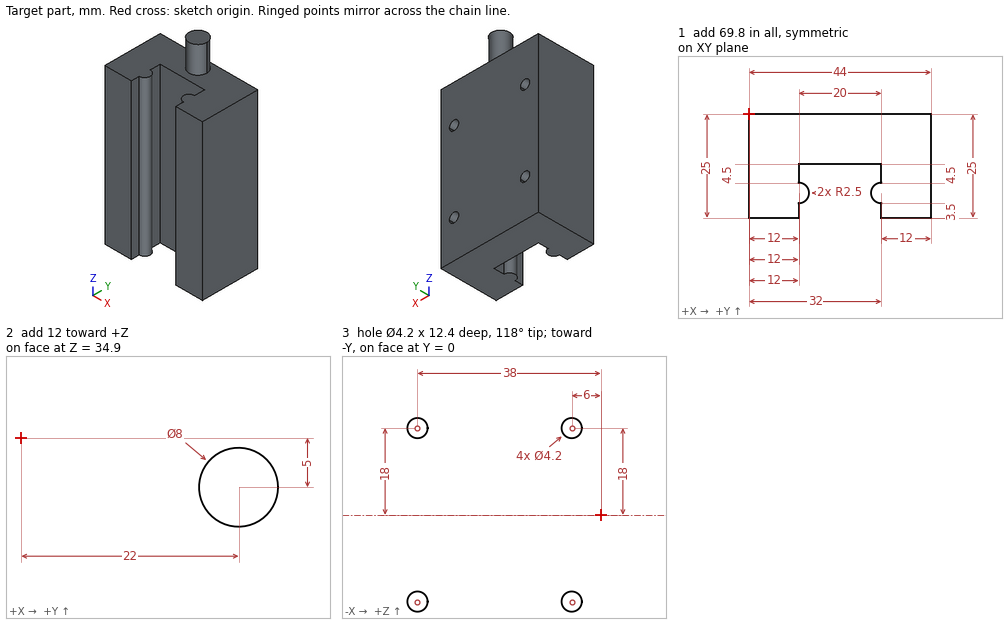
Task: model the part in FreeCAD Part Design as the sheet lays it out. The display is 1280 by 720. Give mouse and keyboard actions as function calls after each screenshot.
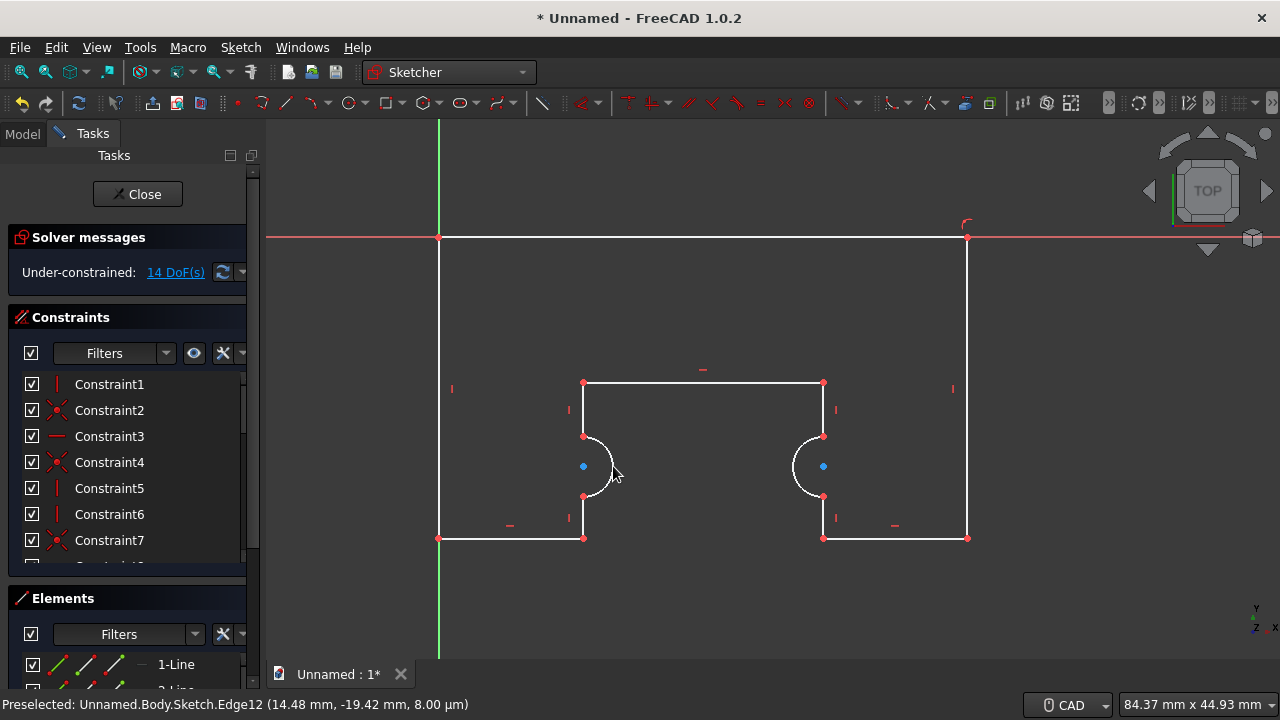
click(799, 449)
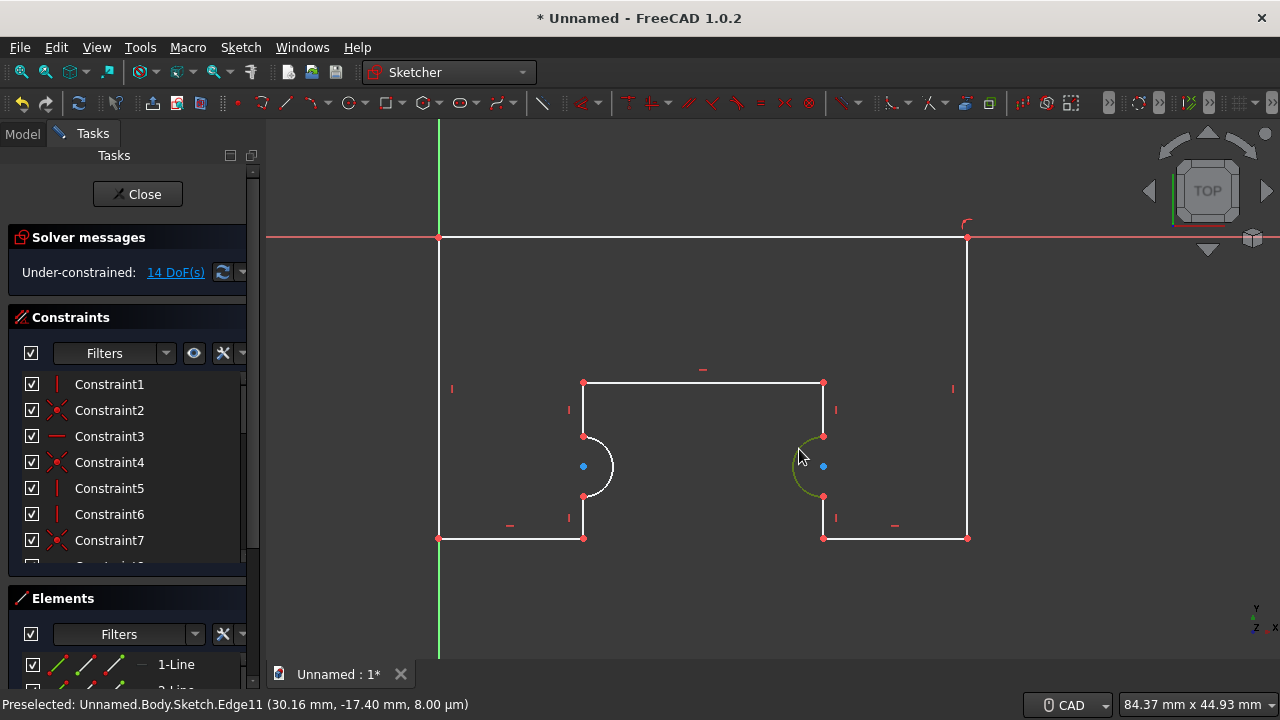
click(607, 485)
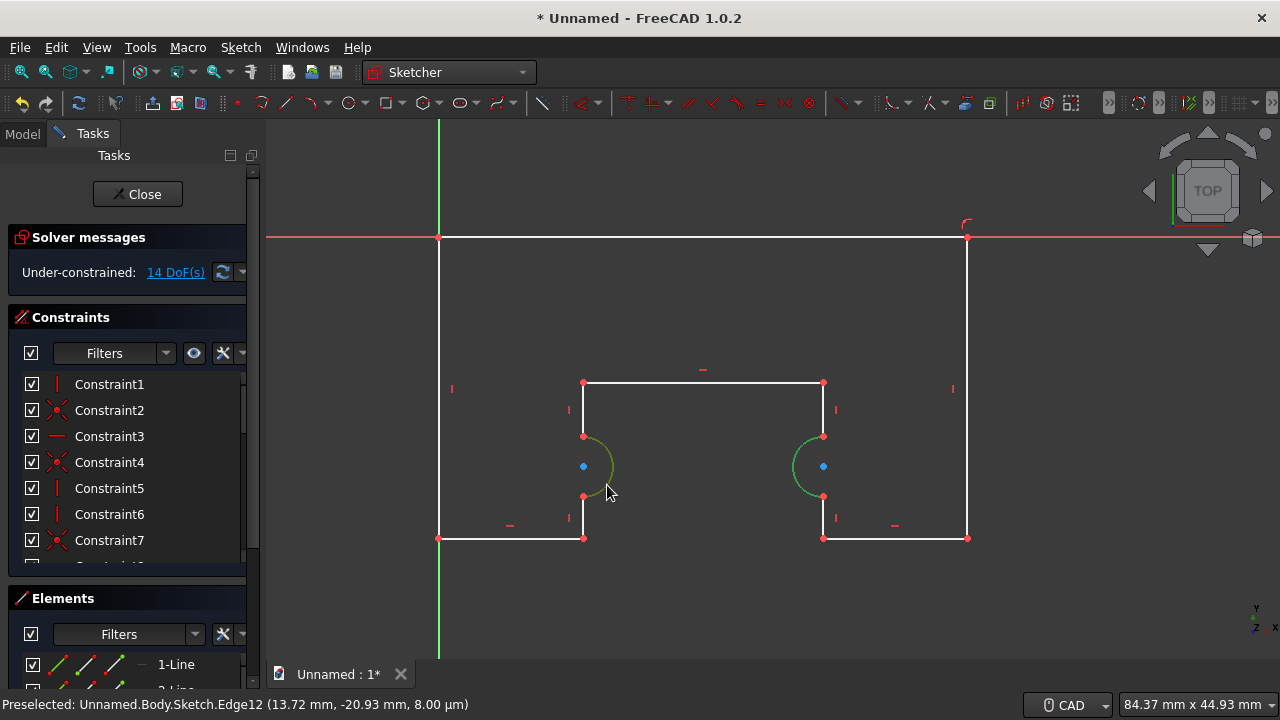
click(762, 104)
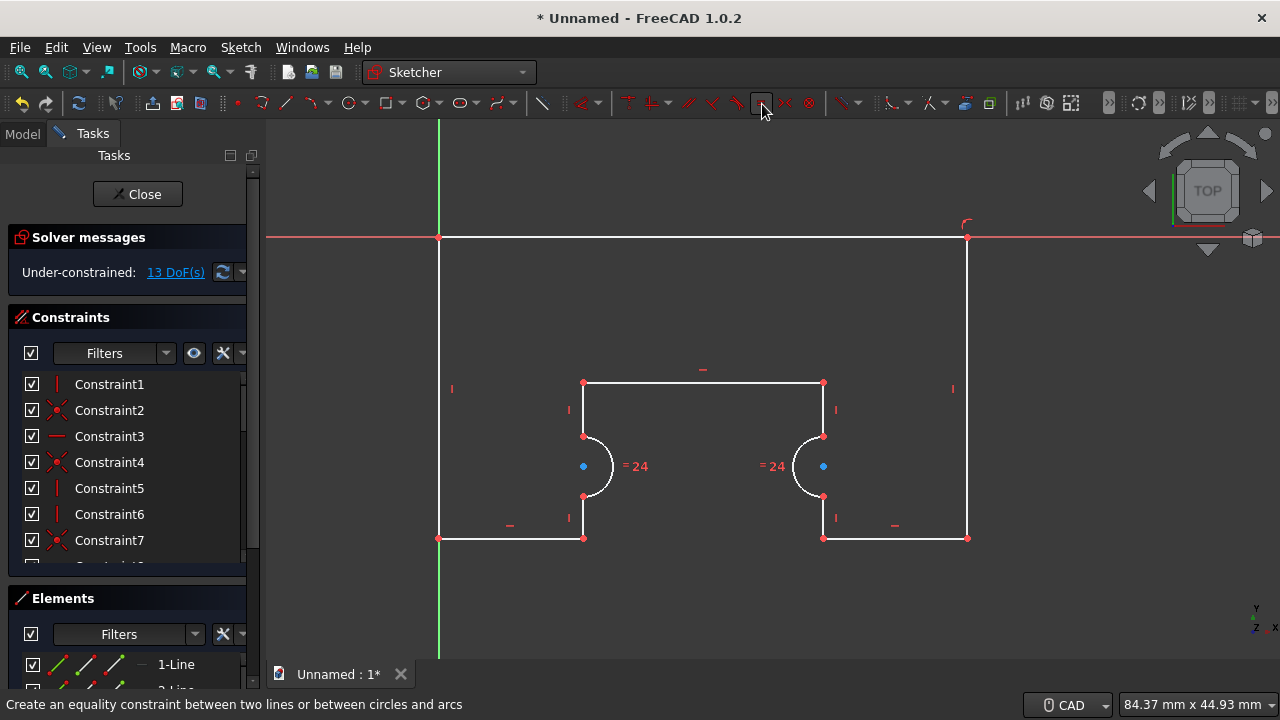
scroll(799, 449, up, 2)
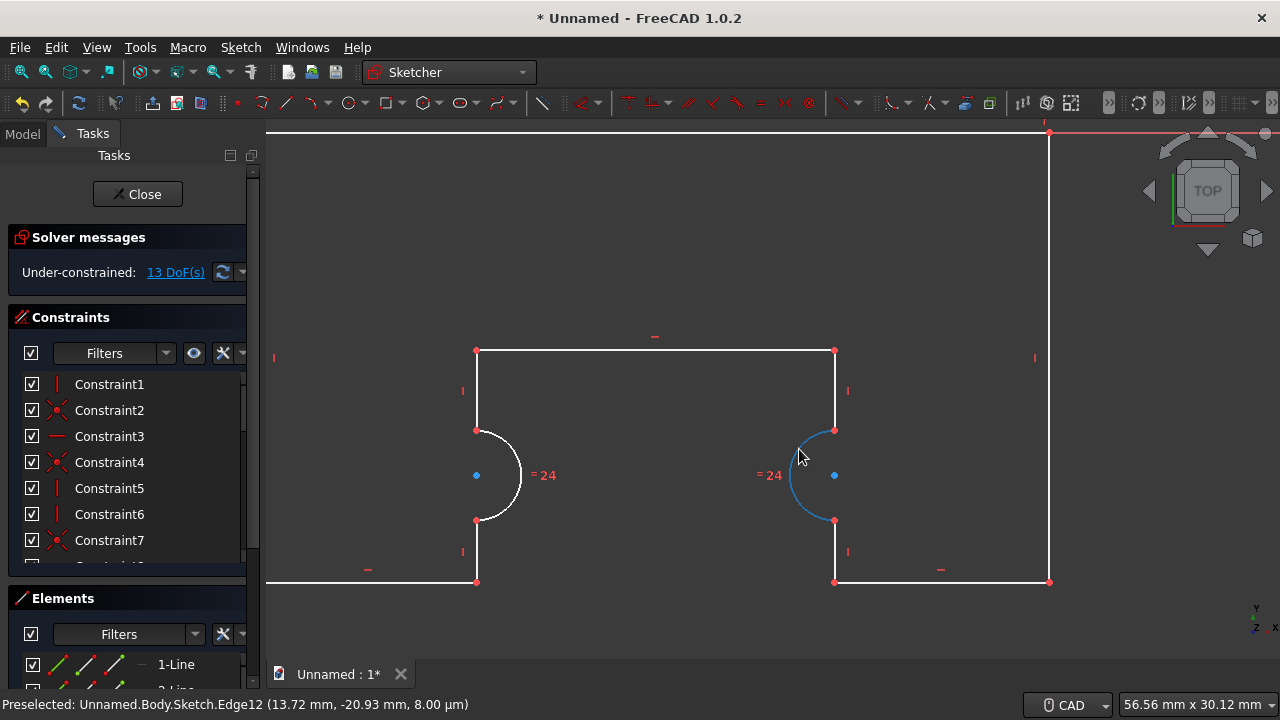
click(798, 449)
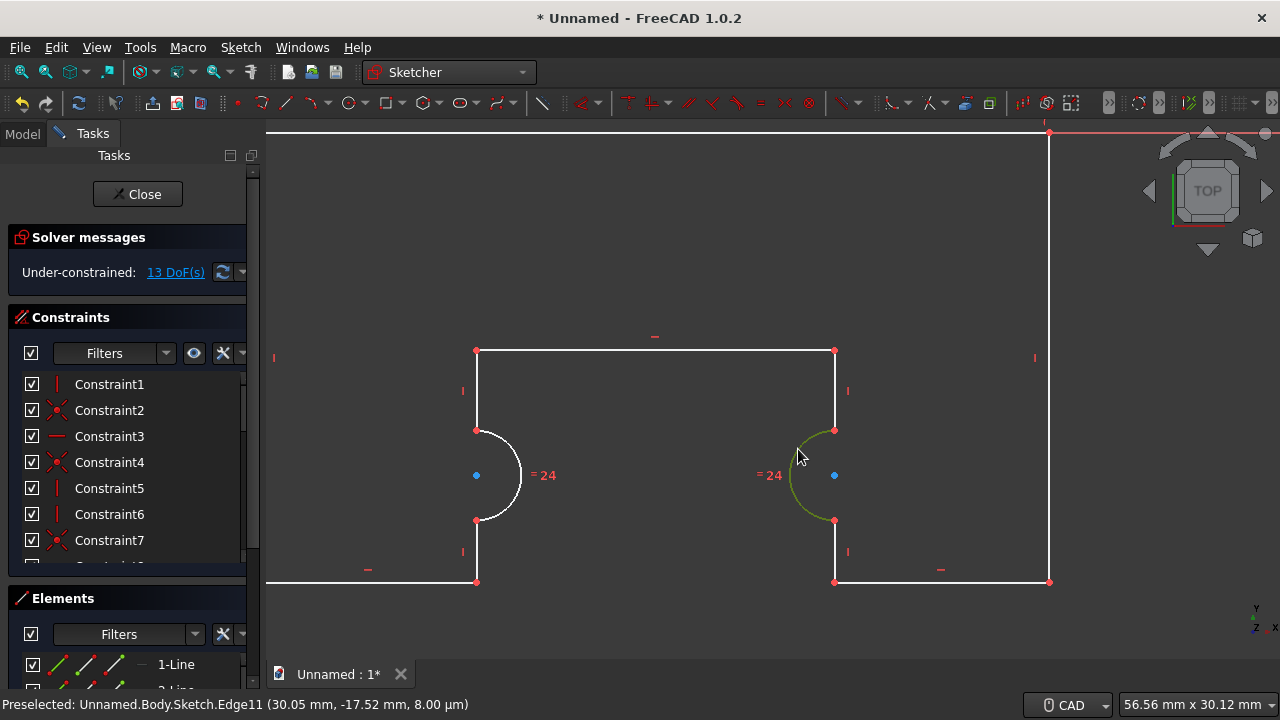
key(k)
key(r)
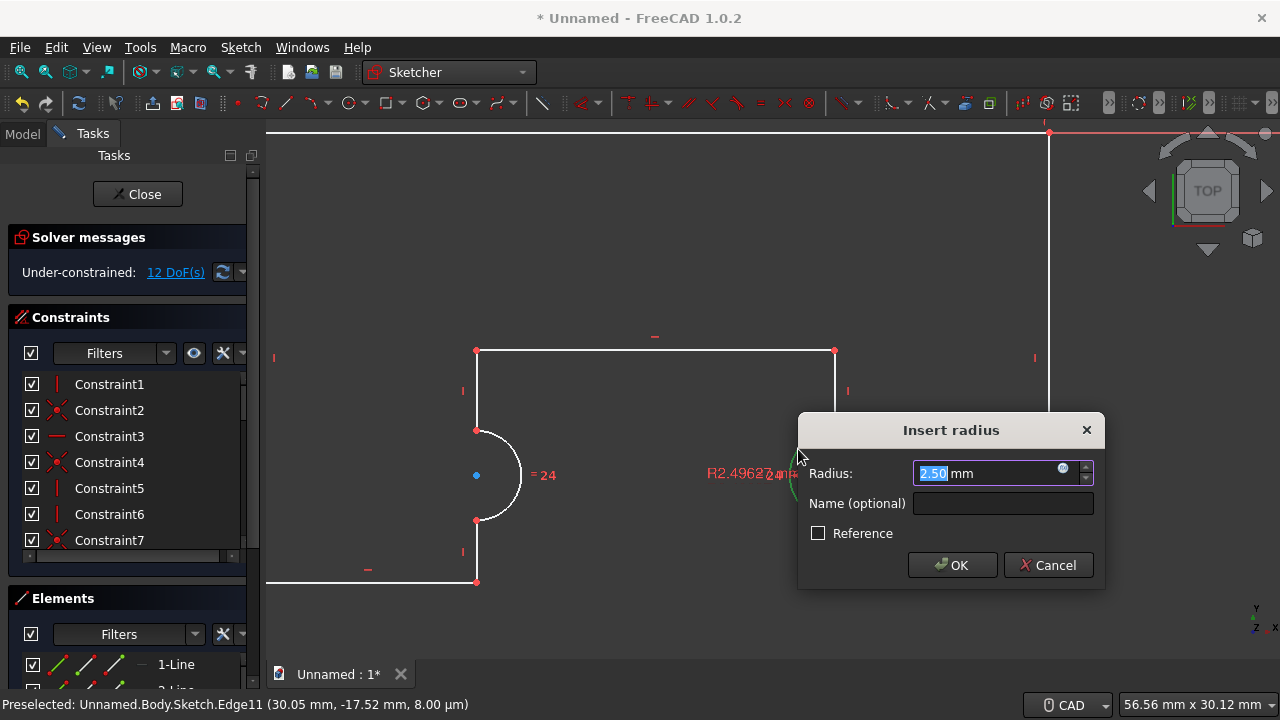
text(2.5)
key(Return)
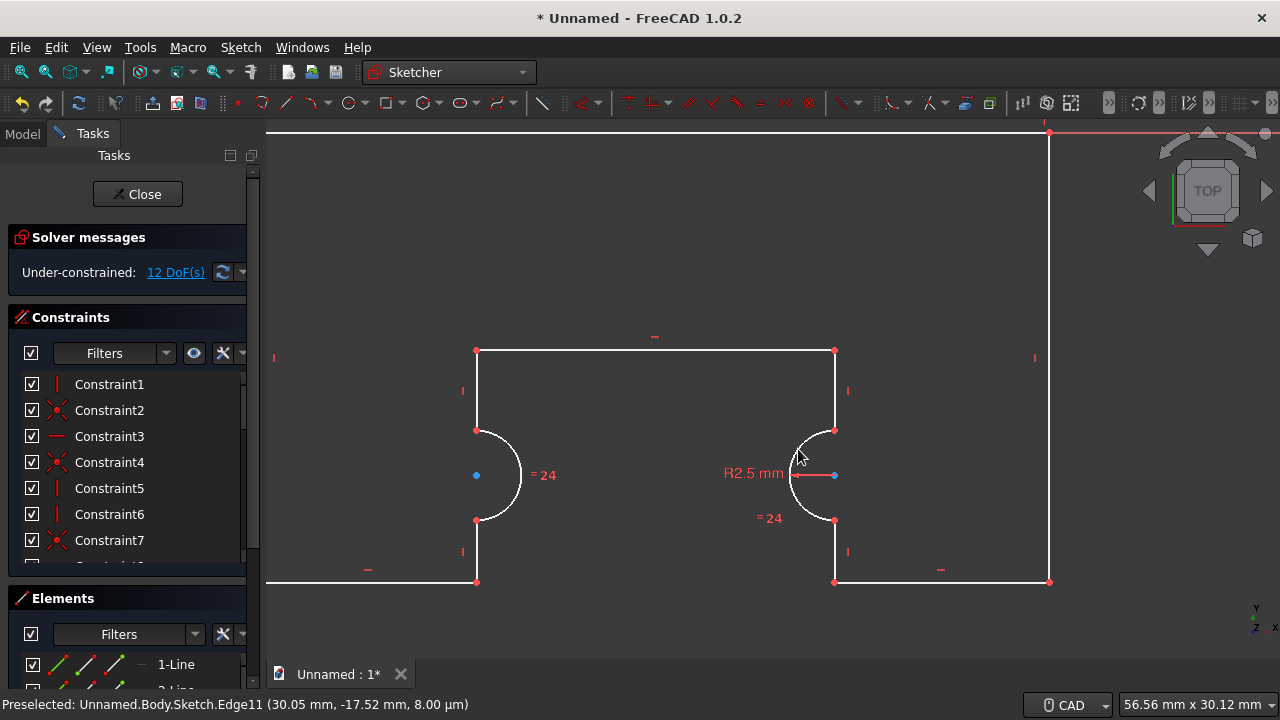
click(584, 350)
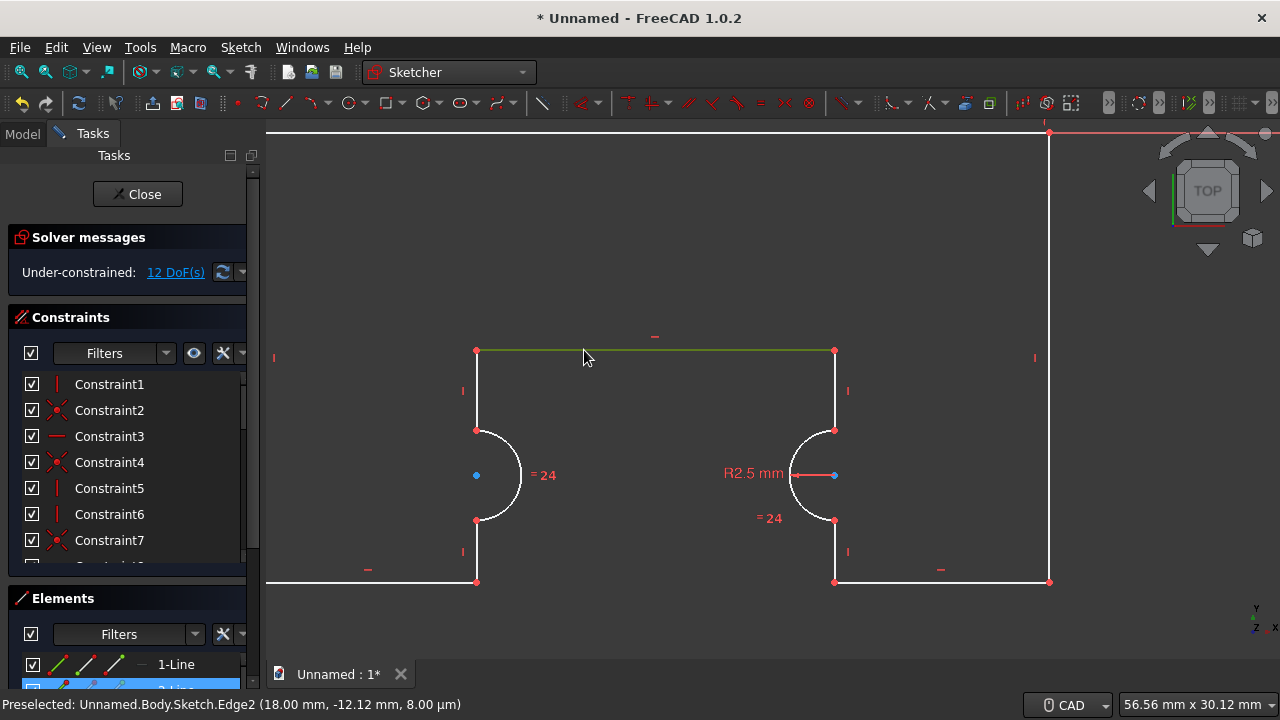
key(l)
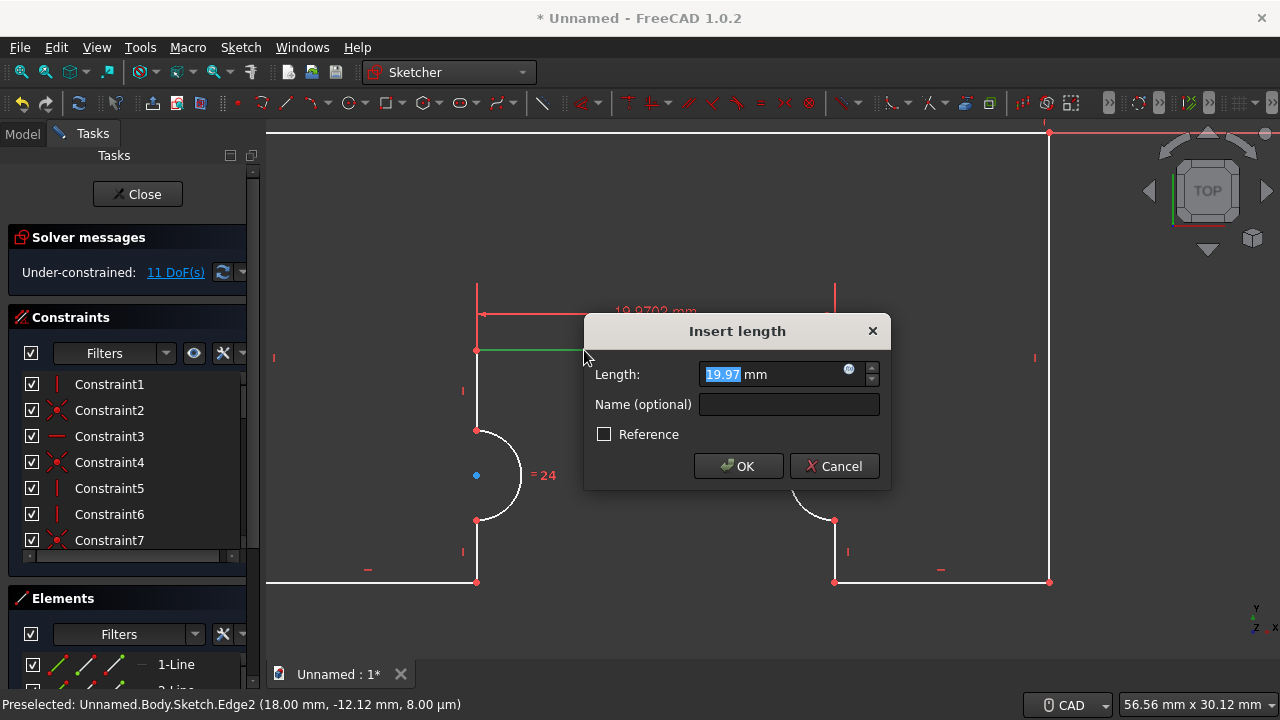
text(20)
key(Return)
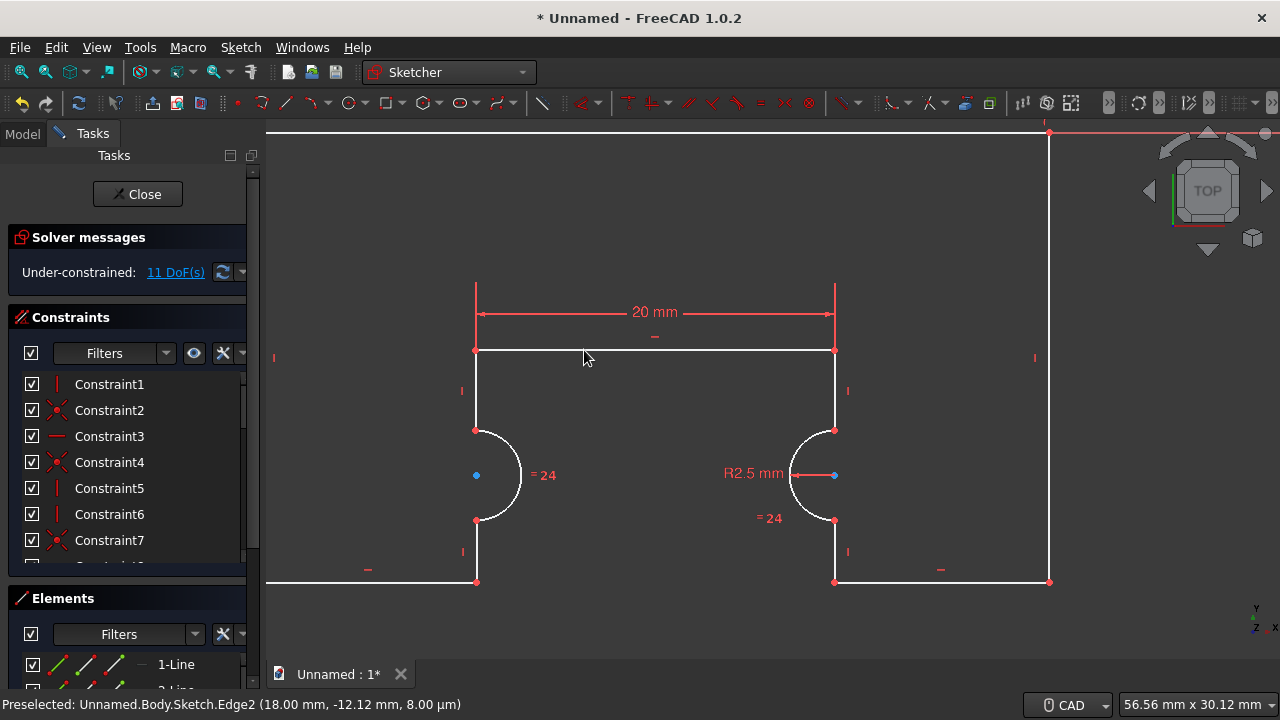
click(899, 583)